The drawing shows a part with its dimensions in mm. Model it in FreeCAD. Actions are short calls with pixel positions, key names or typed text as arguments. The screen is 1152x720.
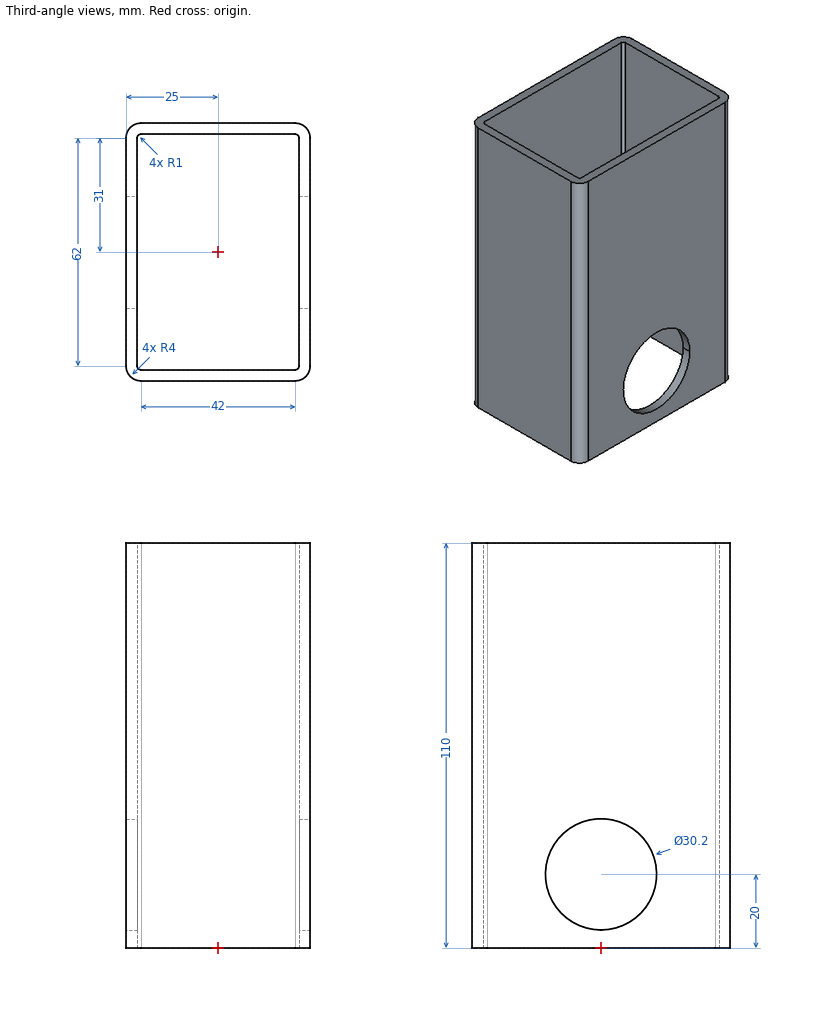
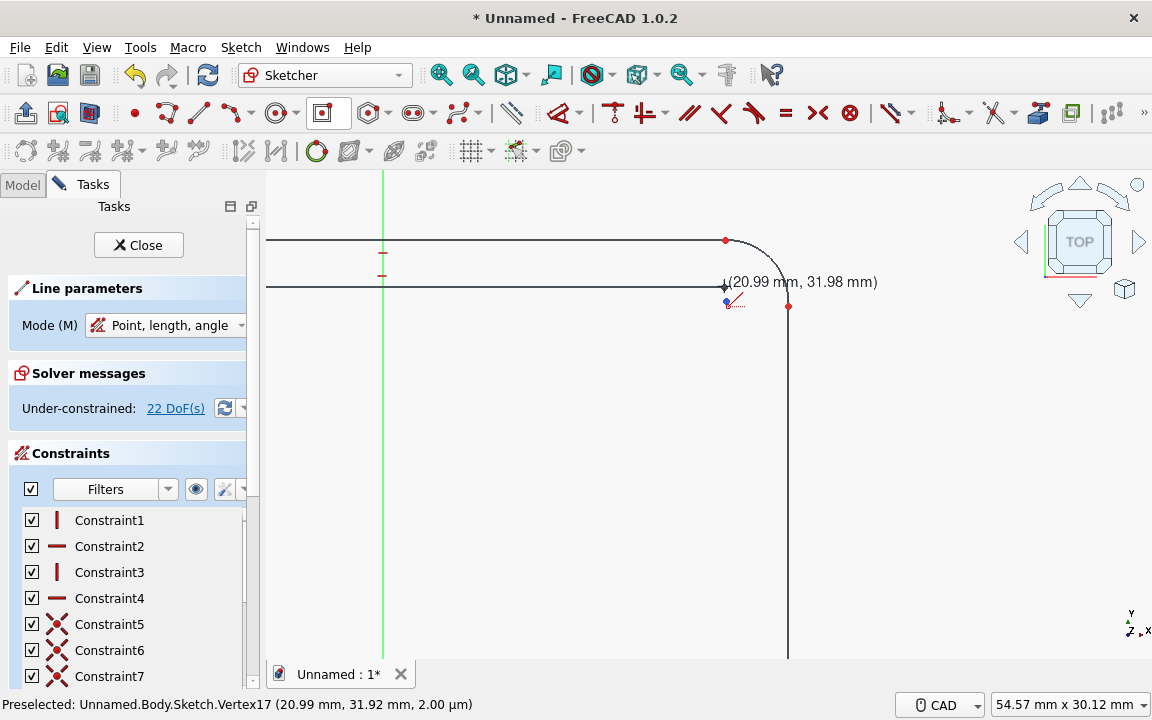
click(740, 303)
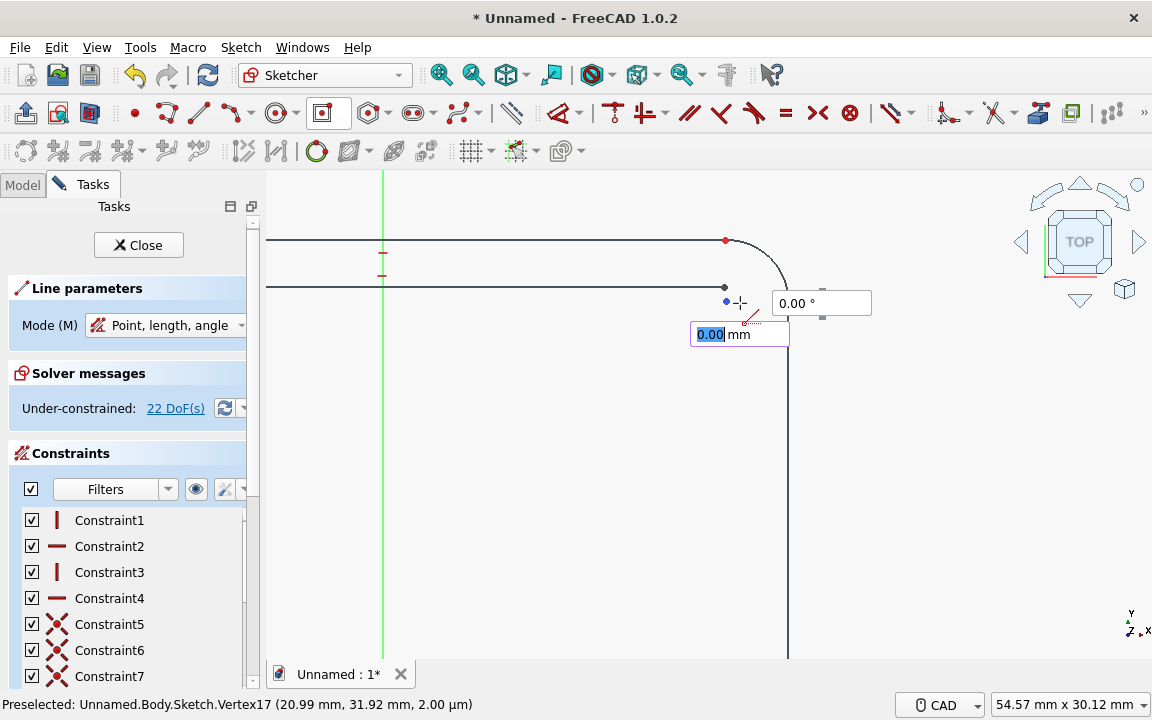
scroll(725, 286, down, 7)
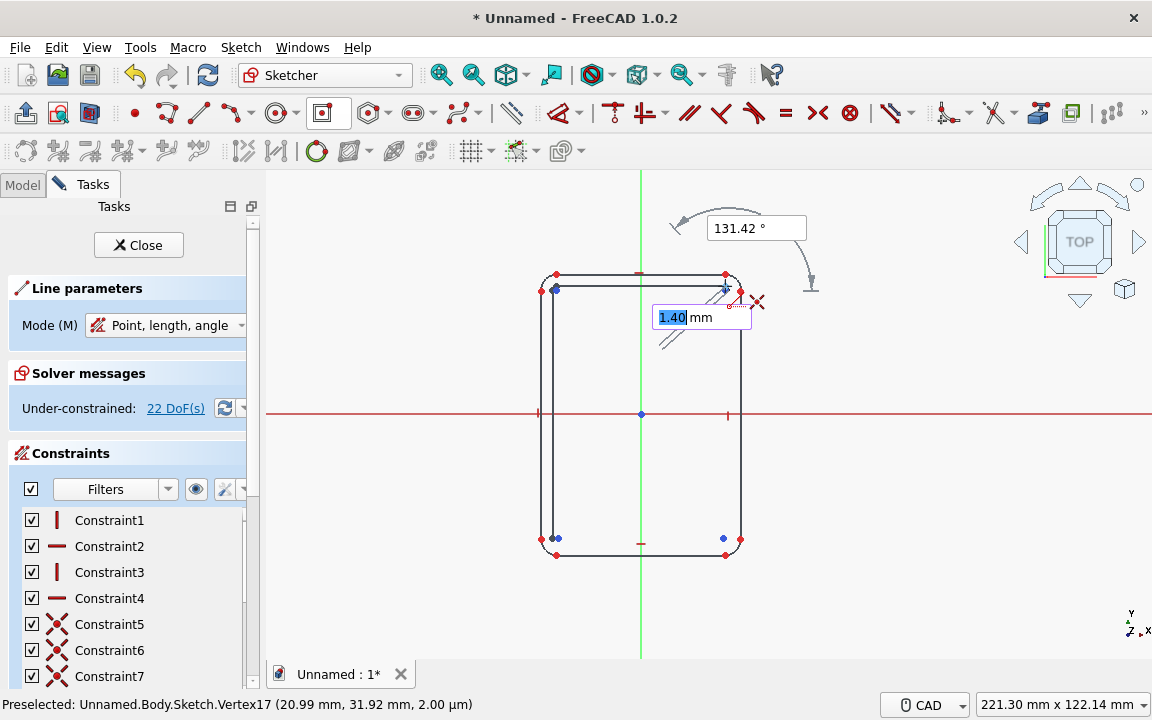
scroll(729, 539, up, 7)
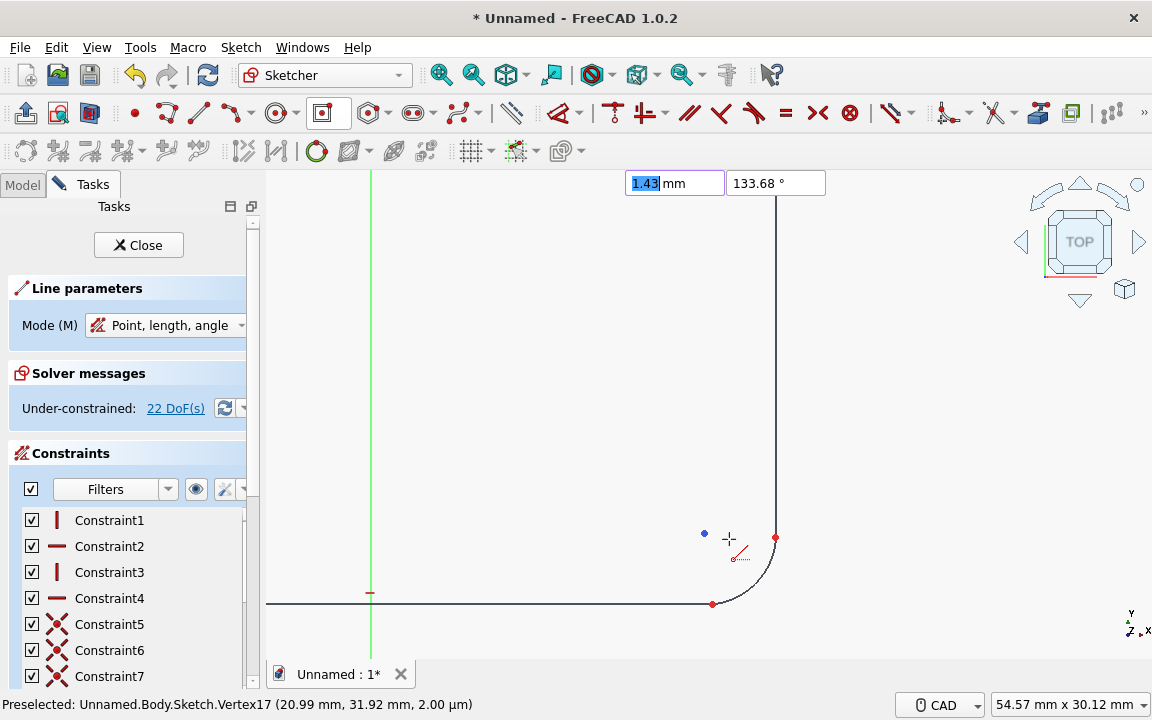
click(728, 535)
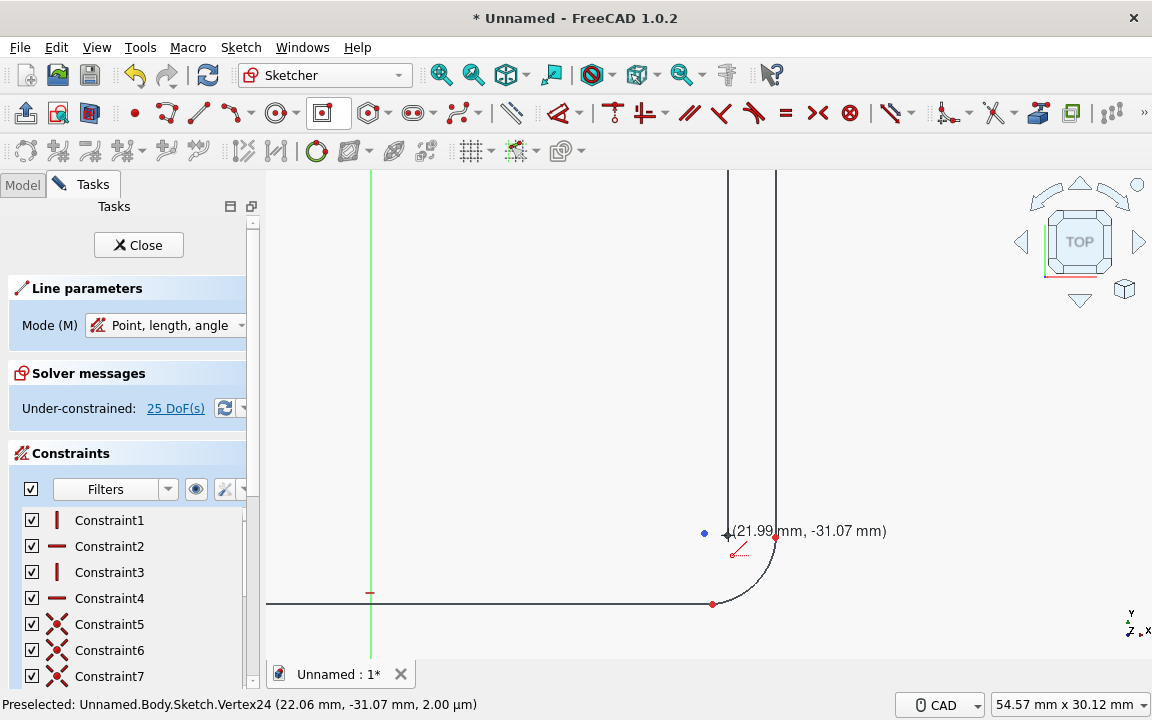
click(712, 551)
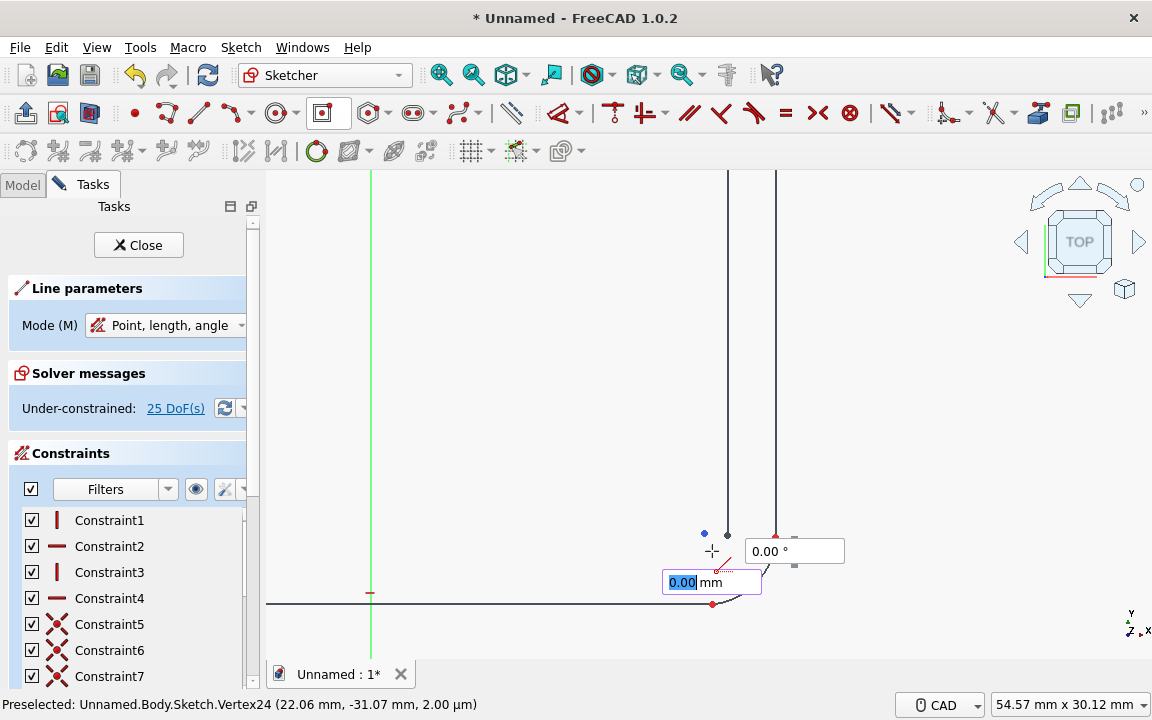
scroll(729, 540, down, 7)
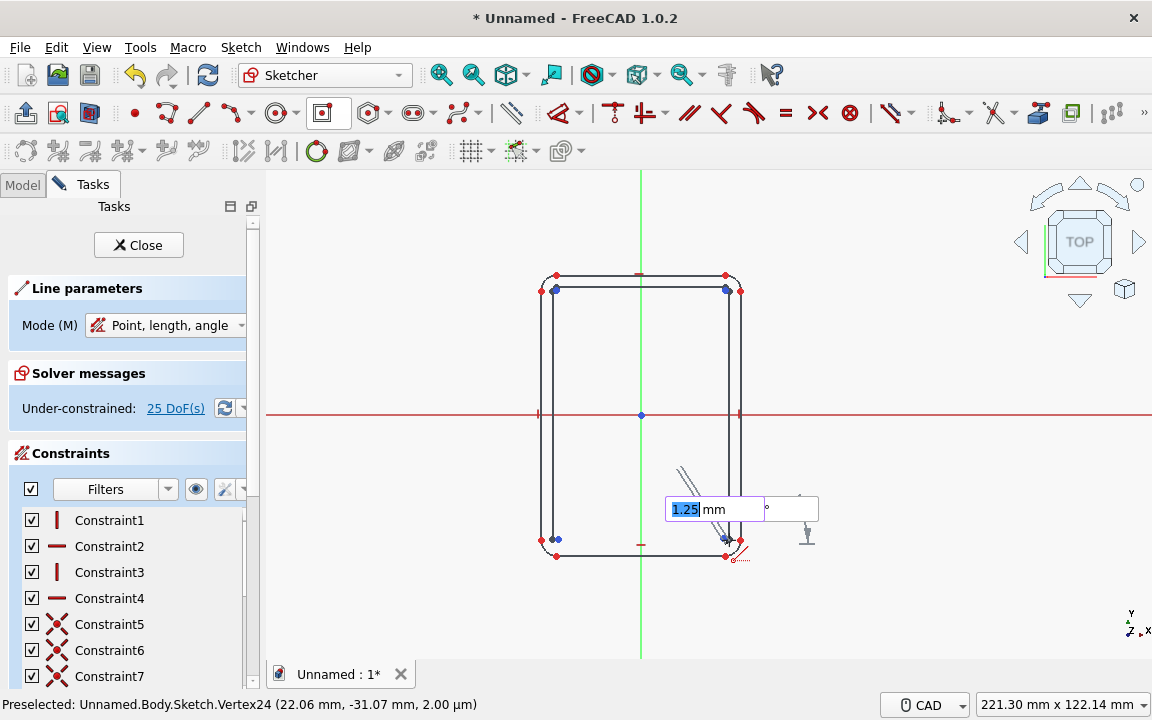
scroll(557, 543, up, 7)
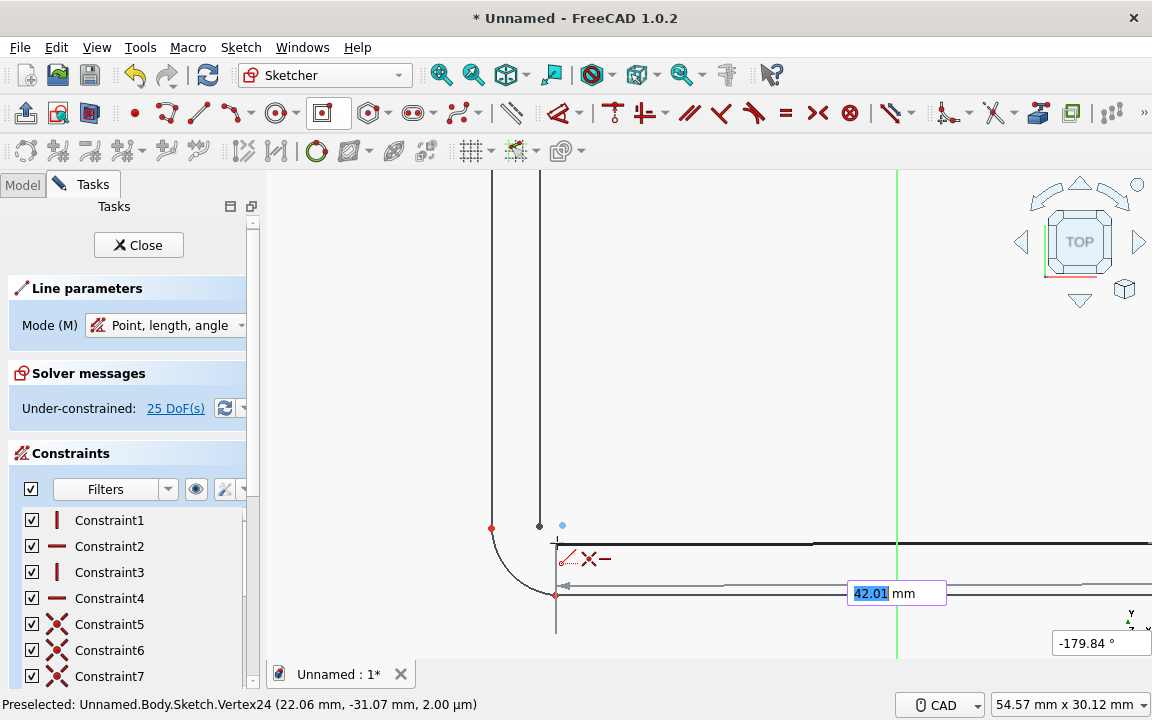
click(556, 542)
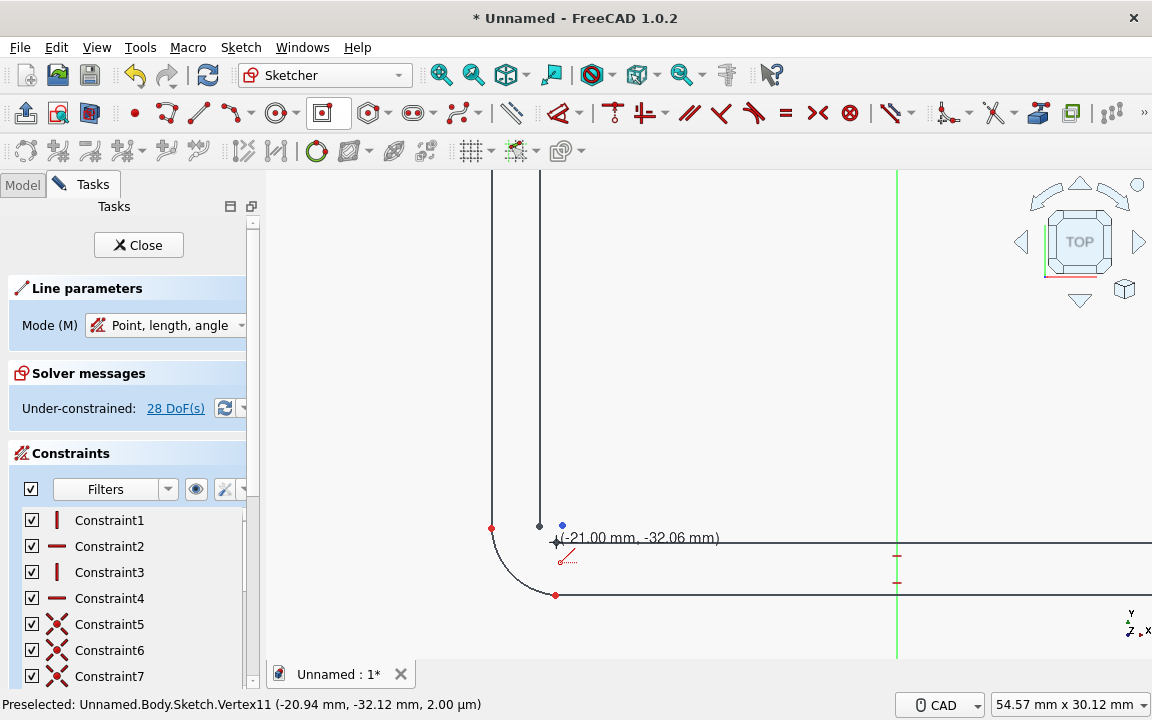
click(232, 114)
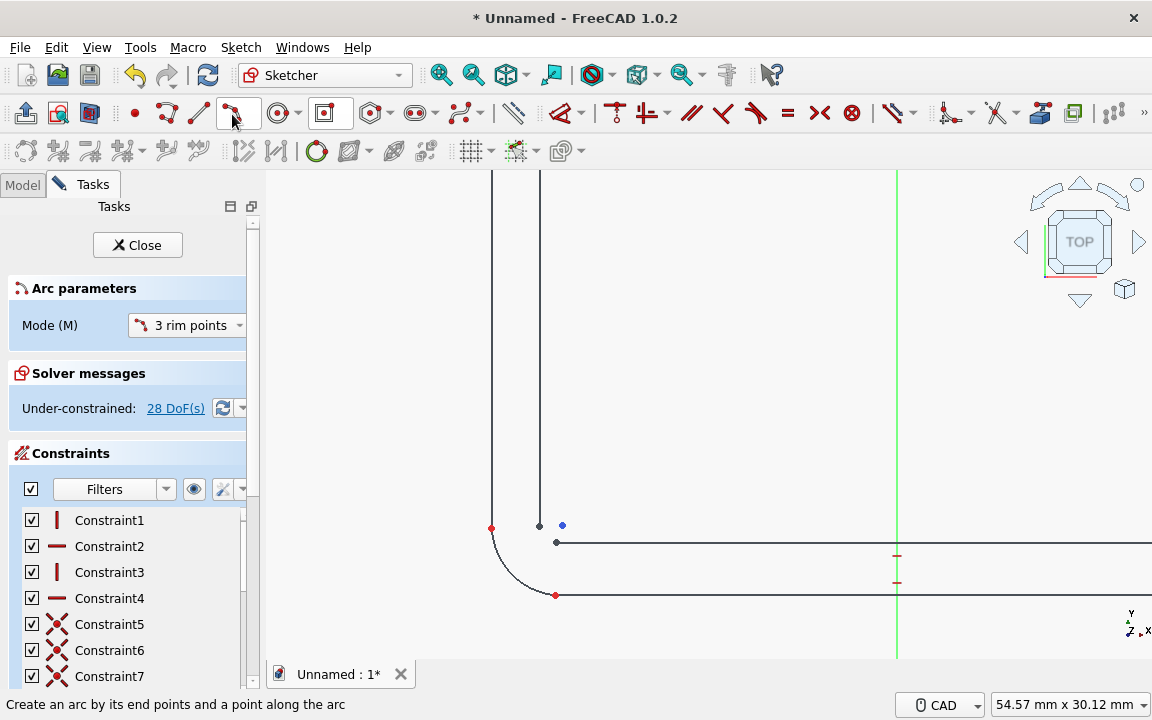
scroll(557, 543, down, 7)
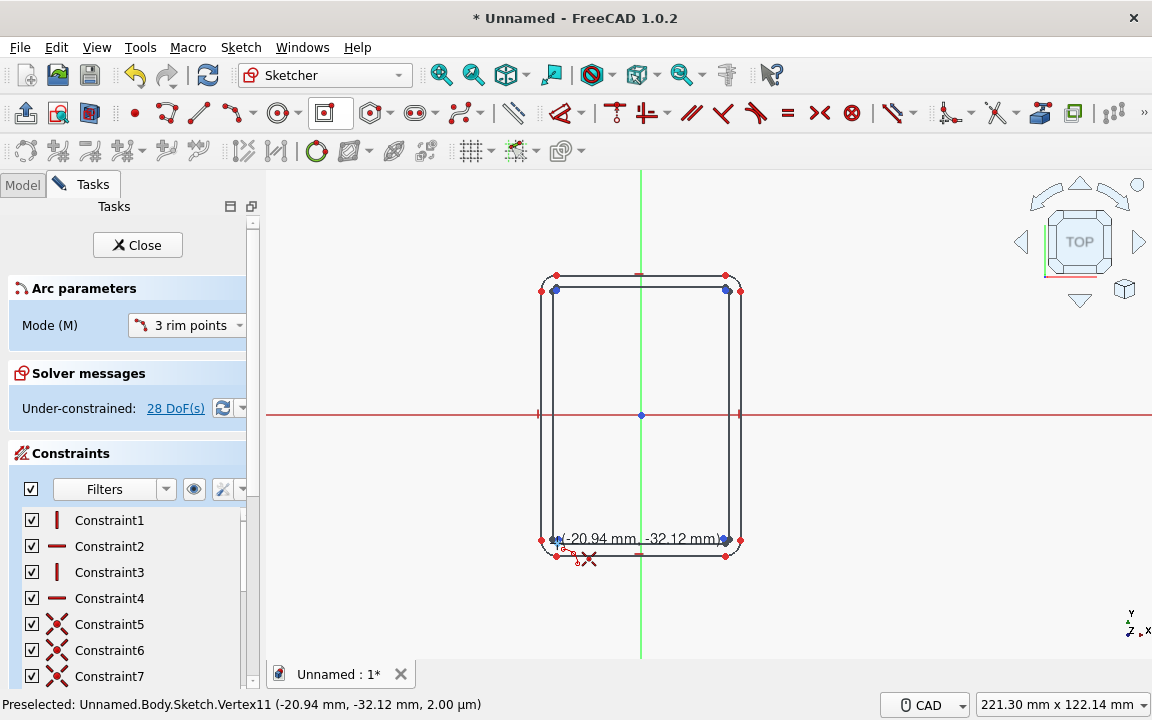
scroll(553, 291, up, 7)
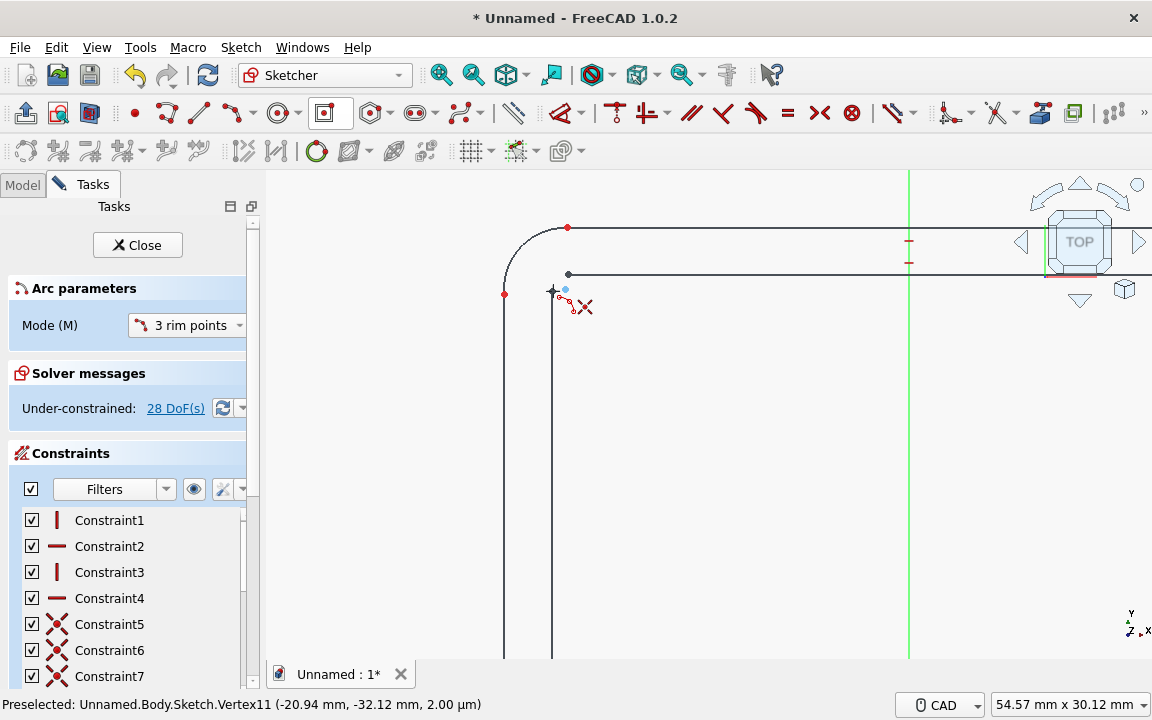
click(552, 292)
click(568, 275)